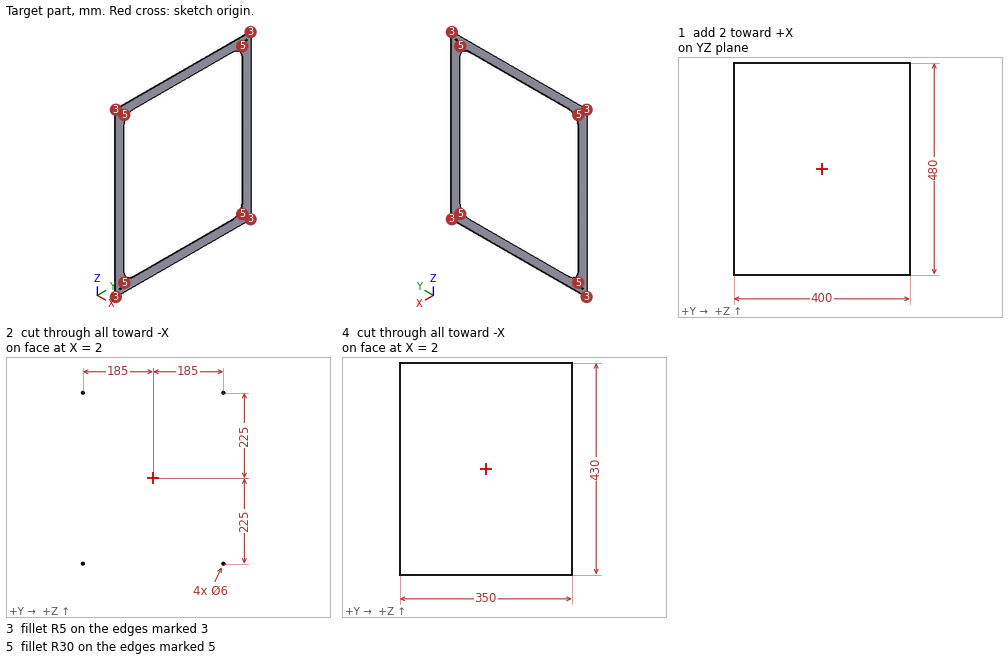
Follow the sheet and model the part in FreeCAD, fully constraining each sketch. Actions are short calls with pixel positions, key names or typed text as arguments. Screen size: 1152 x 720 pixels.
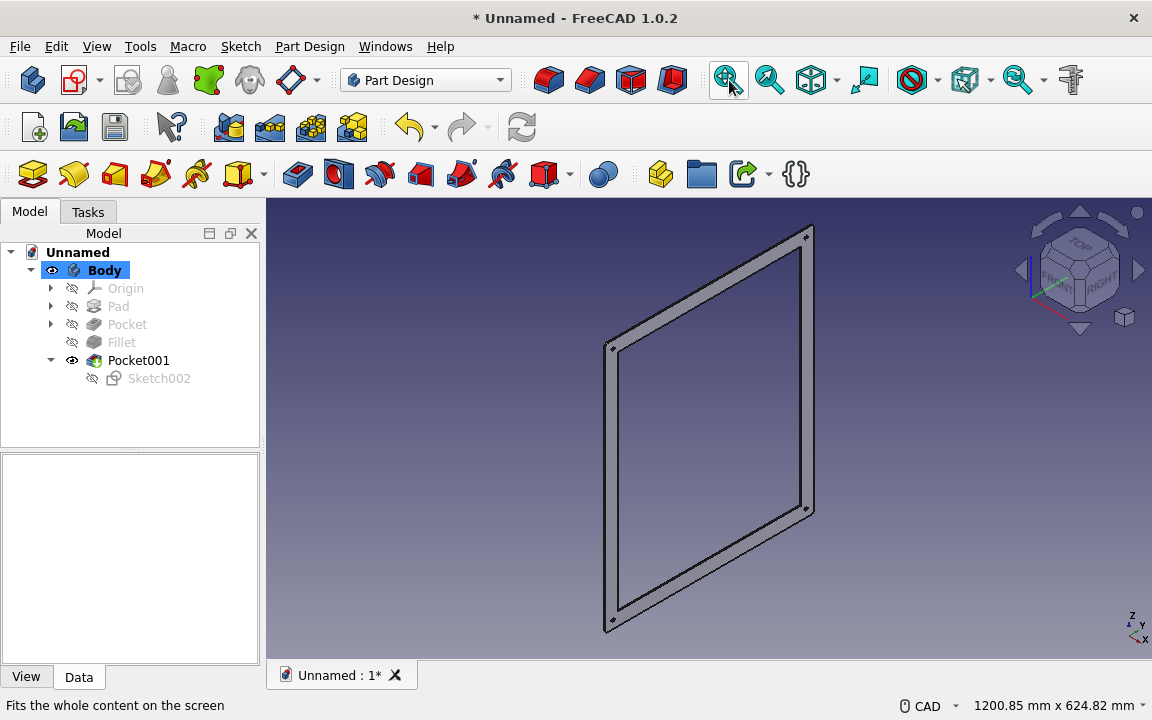
key(1)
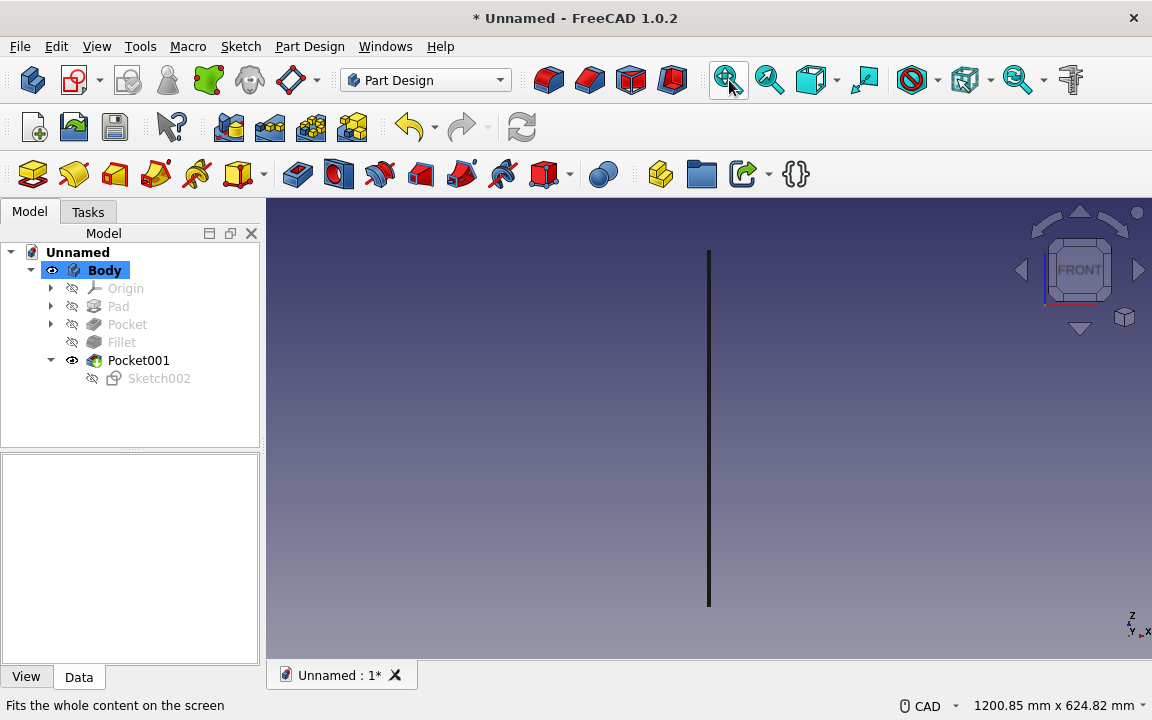
scroll(709, 269, up, 15)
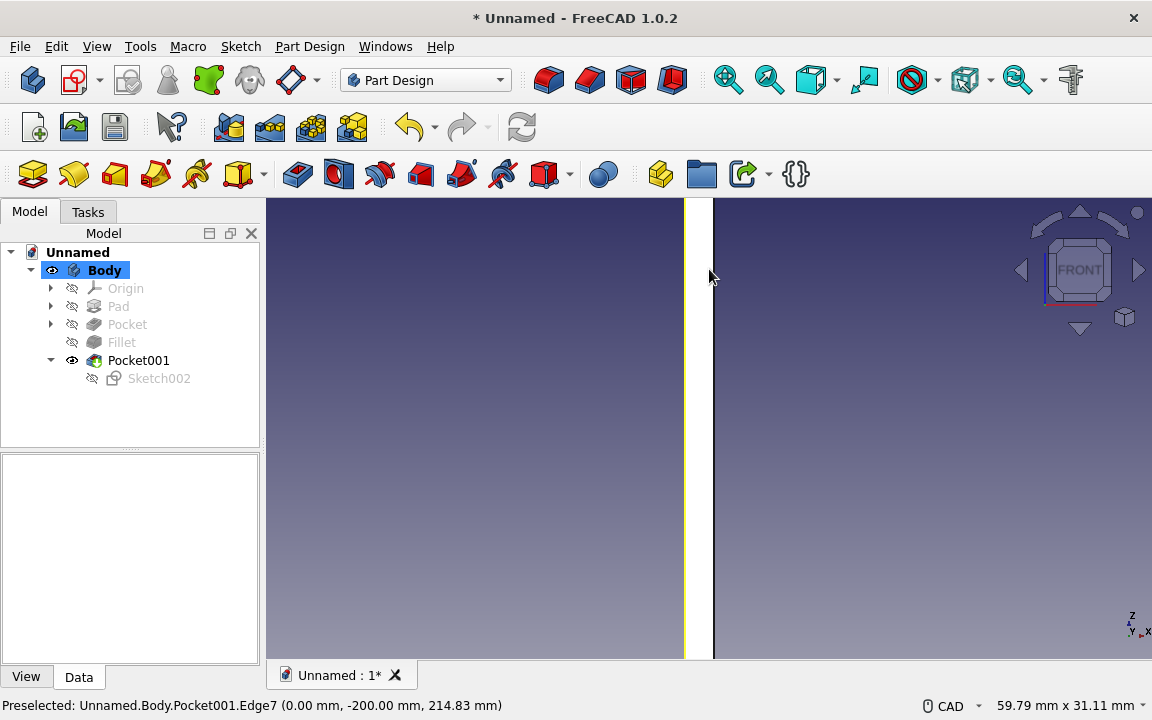
click(729, 80)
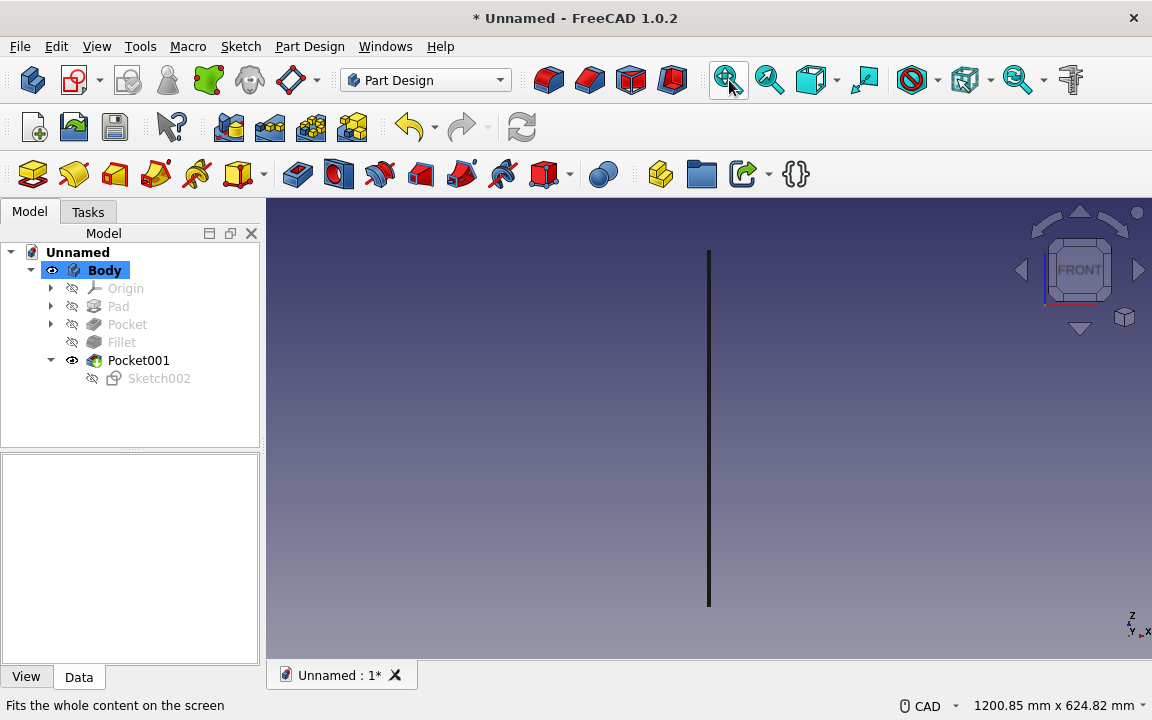
key(3)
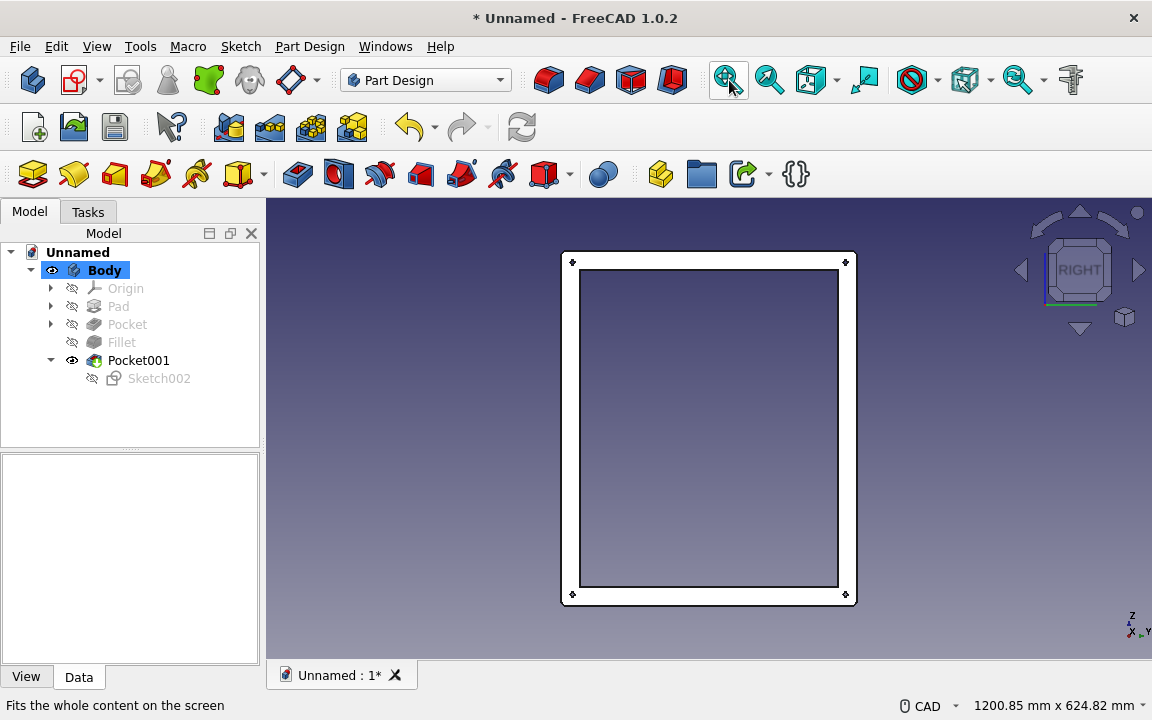
scroll(580, 269, up, 15)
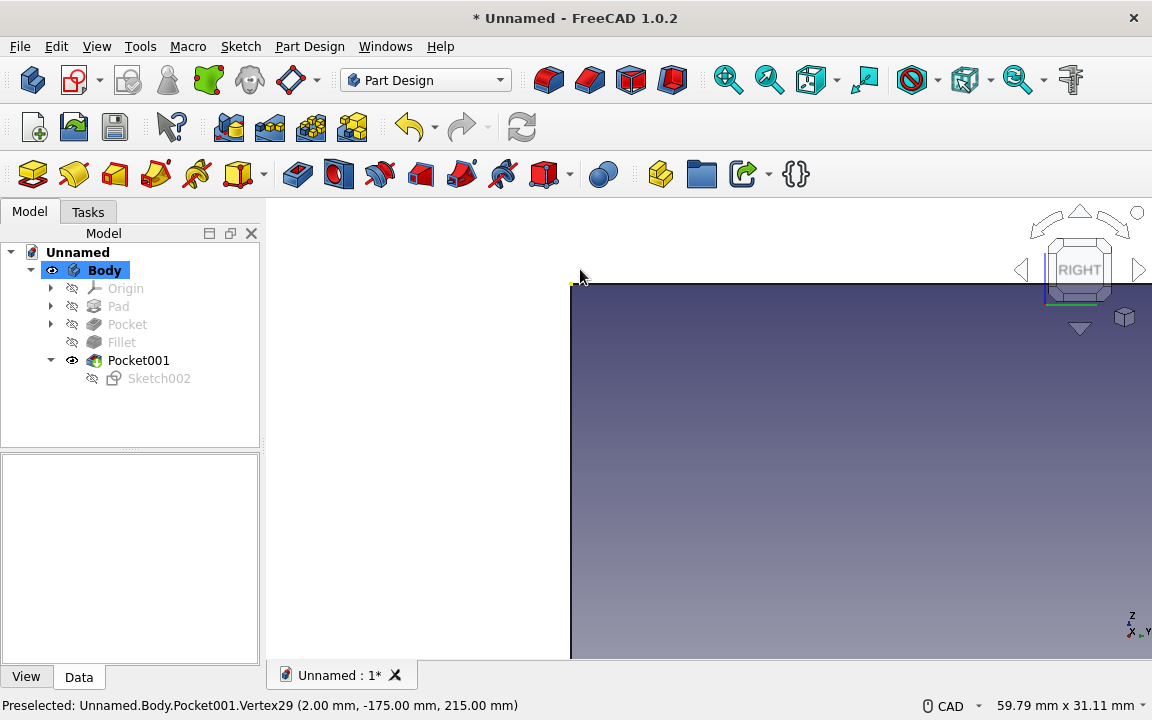
click(729, 80)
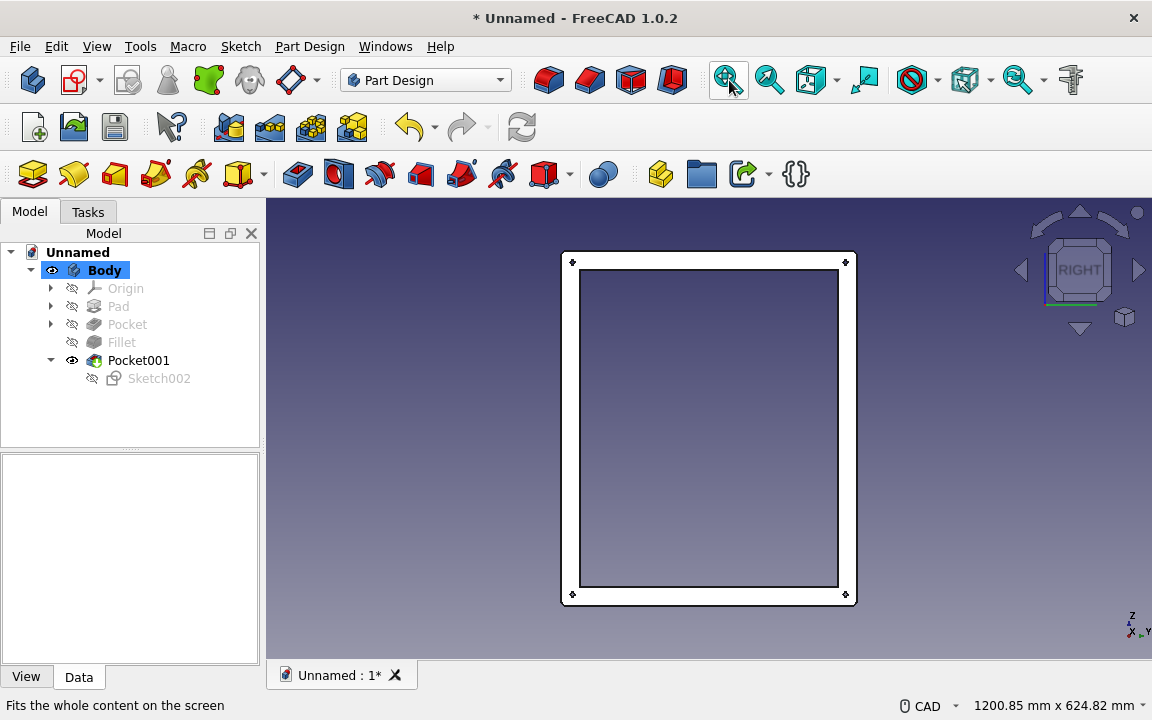
key(5)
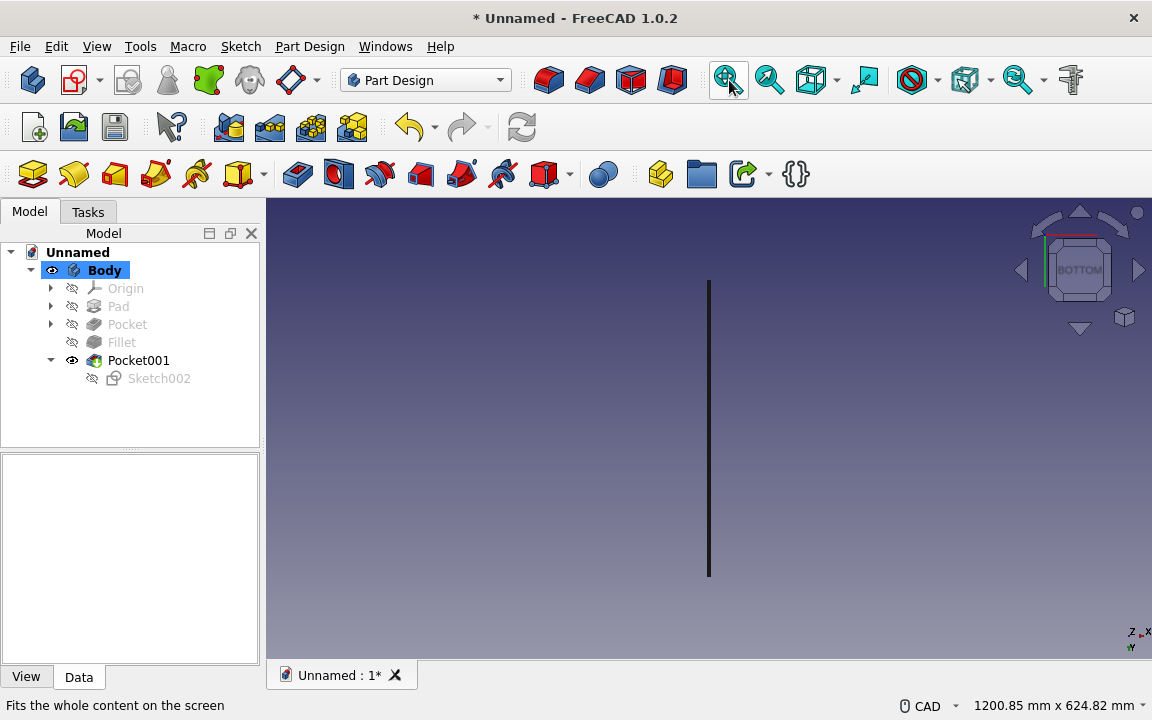
scroll(709, 298, up, 15)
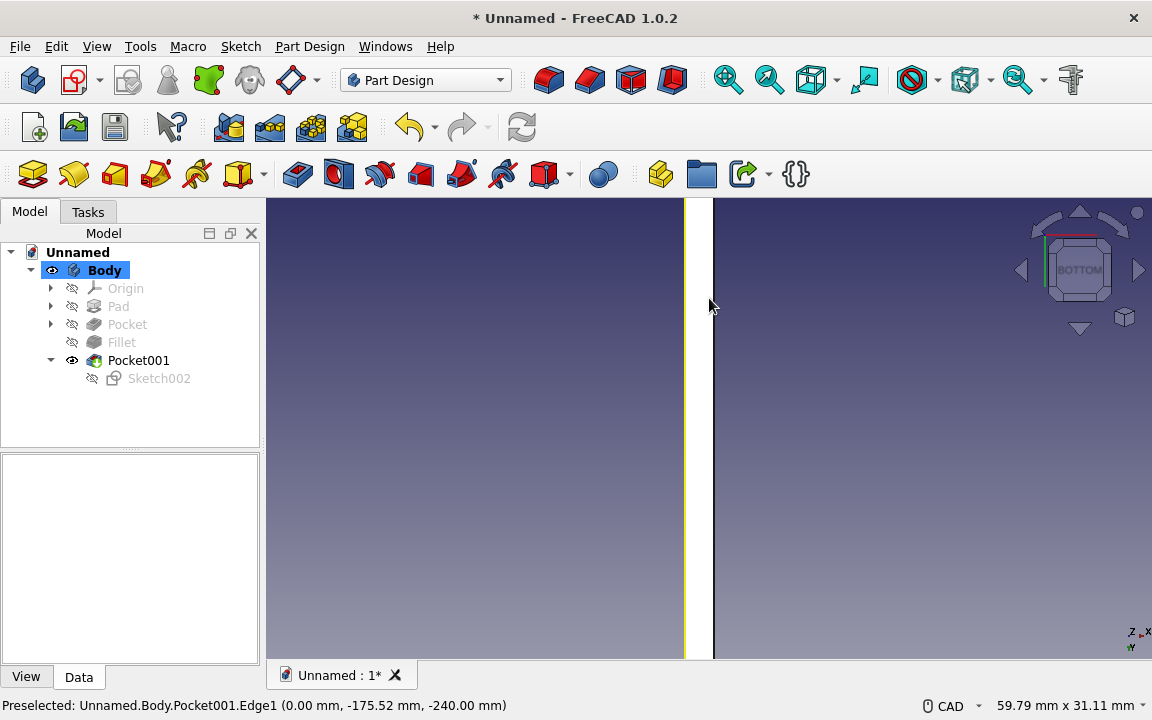
click(729, 80)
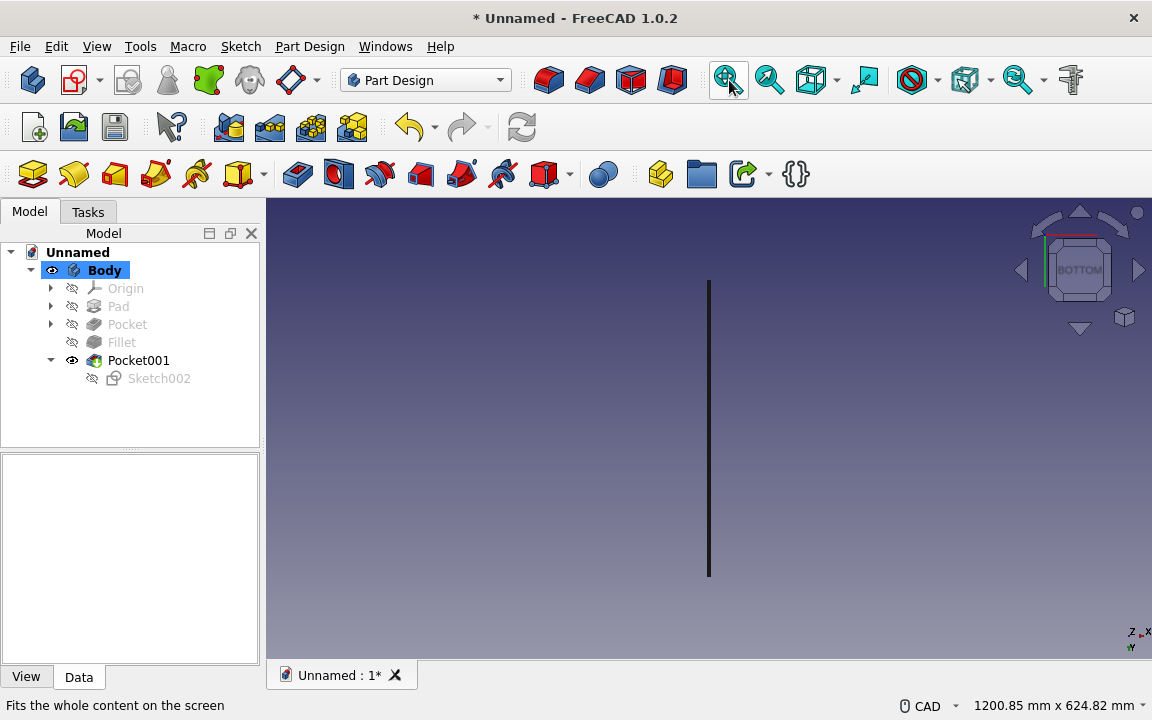
key(4)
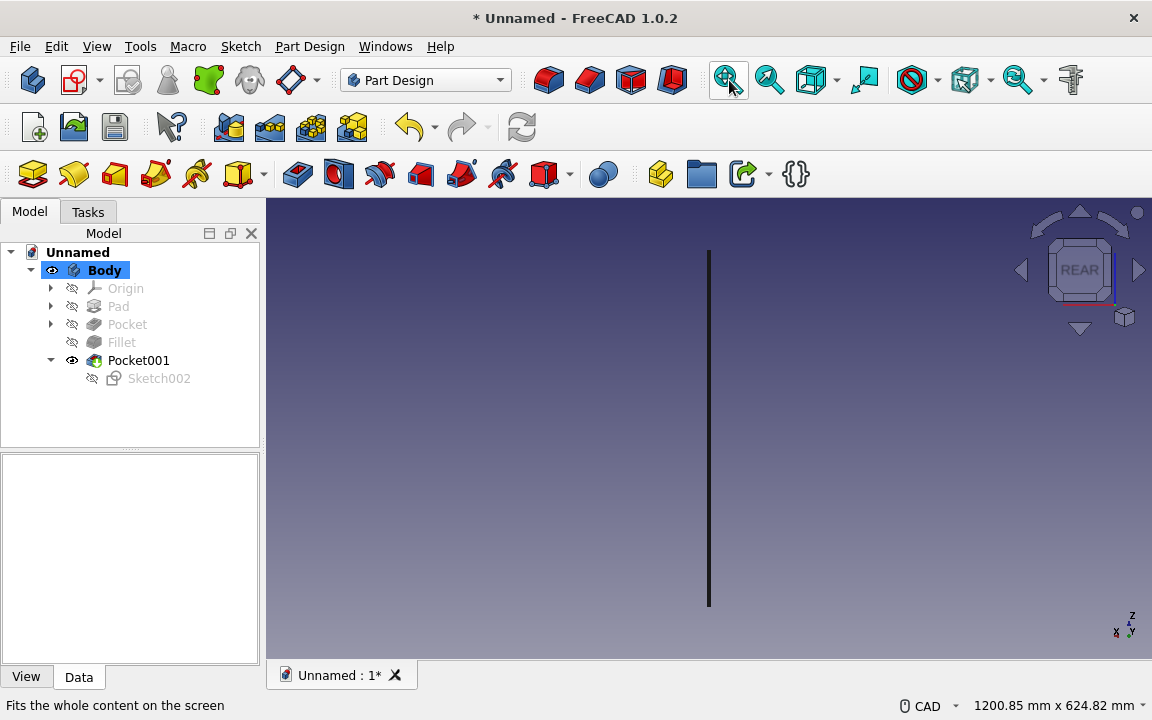
scroll(709, 269, up, 15)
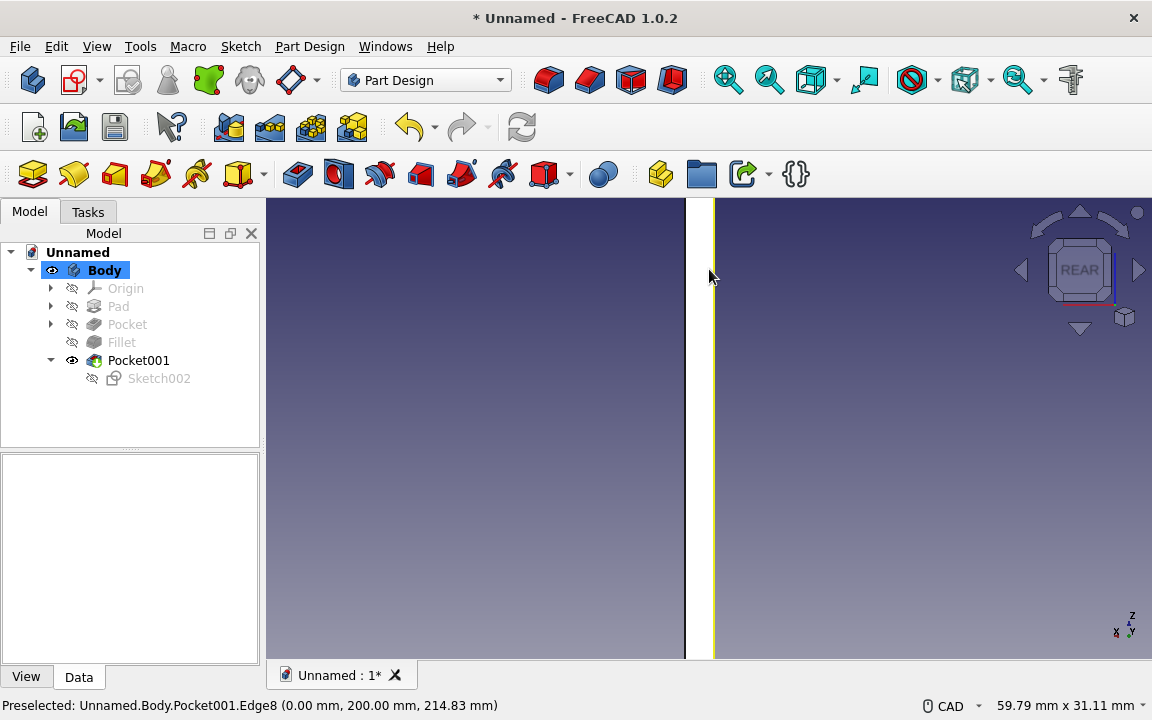
click(729, 80)